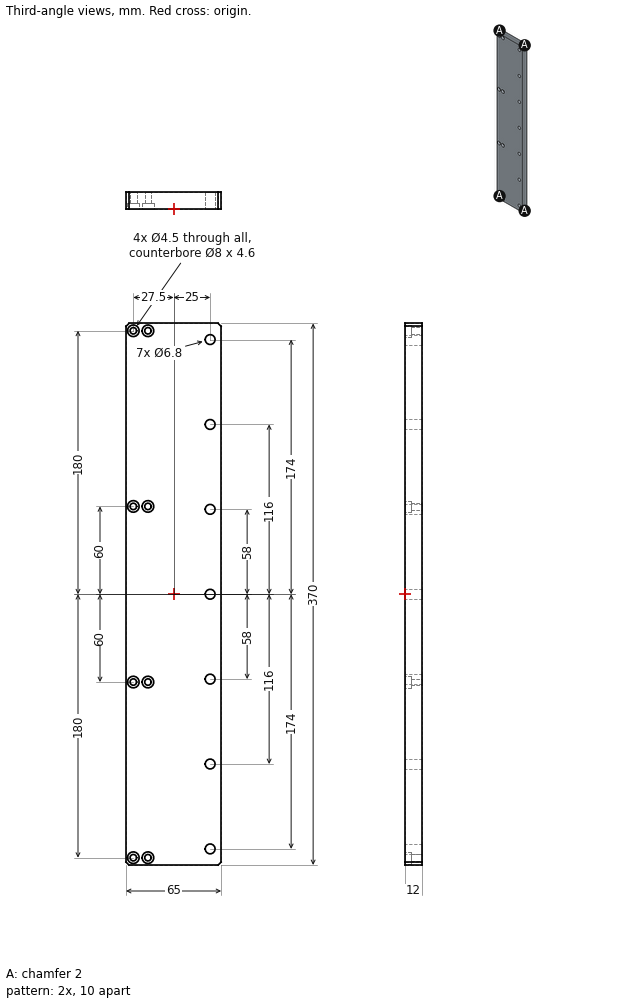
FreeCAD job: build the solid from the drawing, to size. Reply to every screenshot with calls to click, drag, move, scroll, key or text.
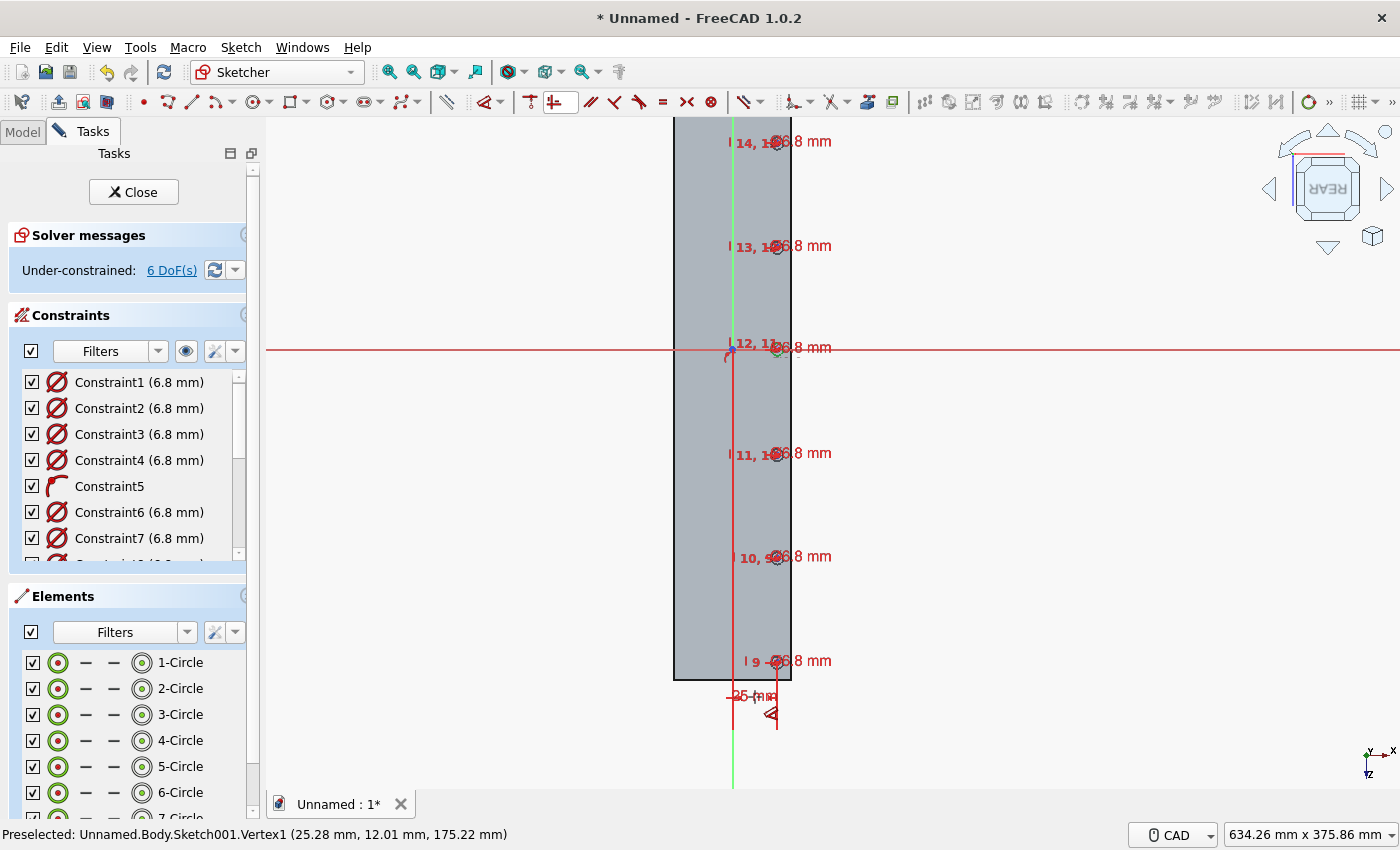
click(777, 455)
click(699, 402)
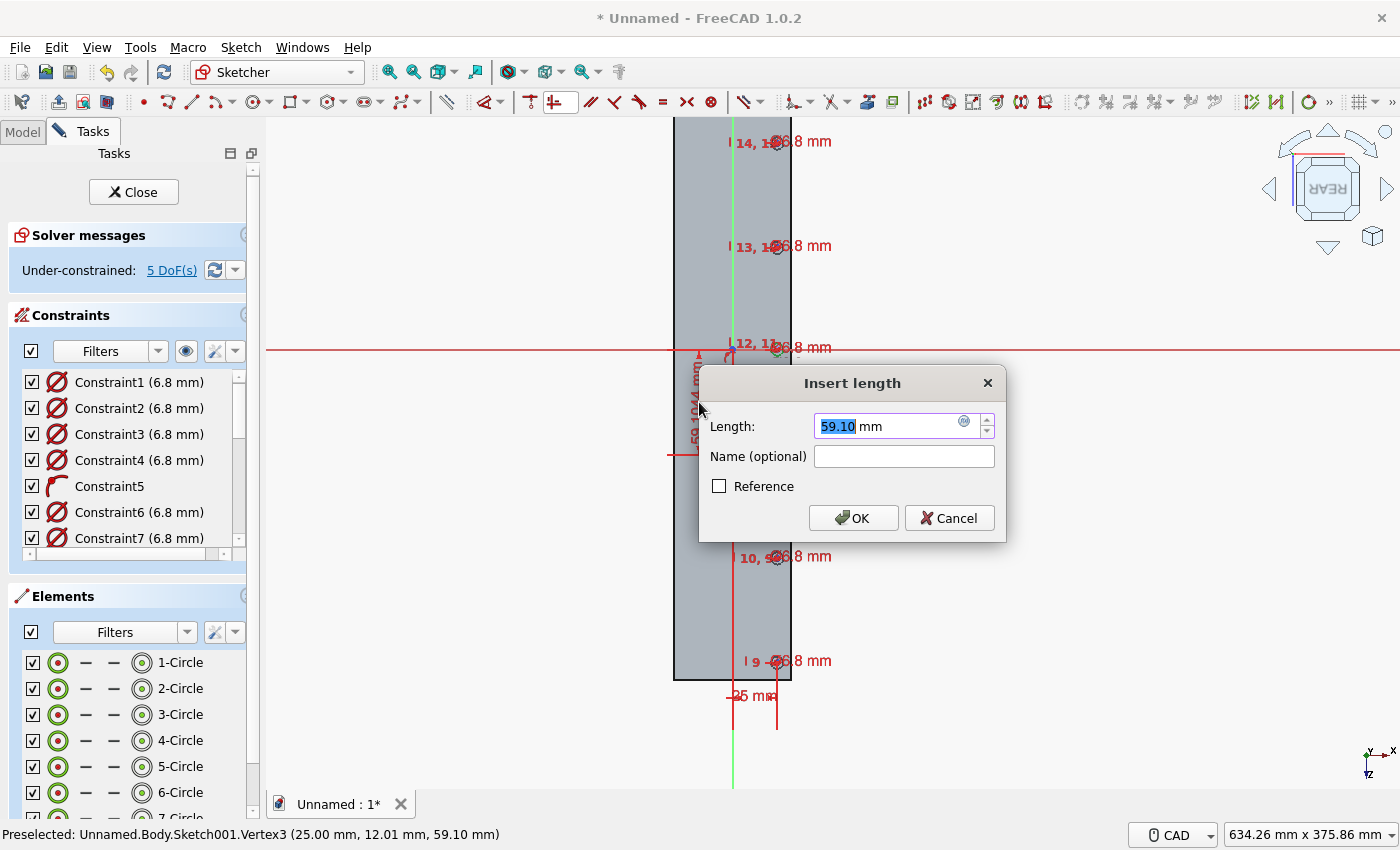
text(58)
key(Return)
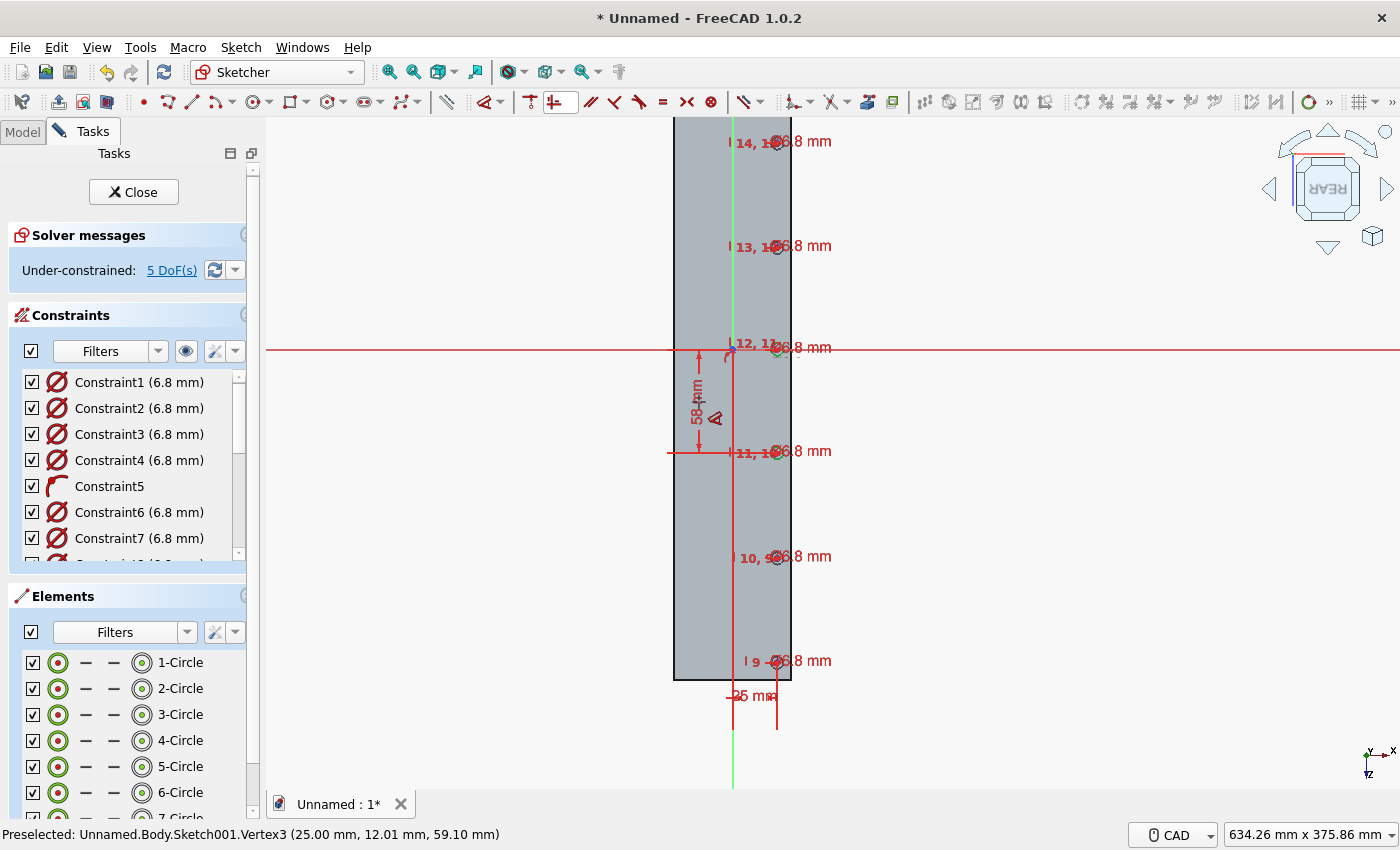
click(777, 248)
click(699, 299)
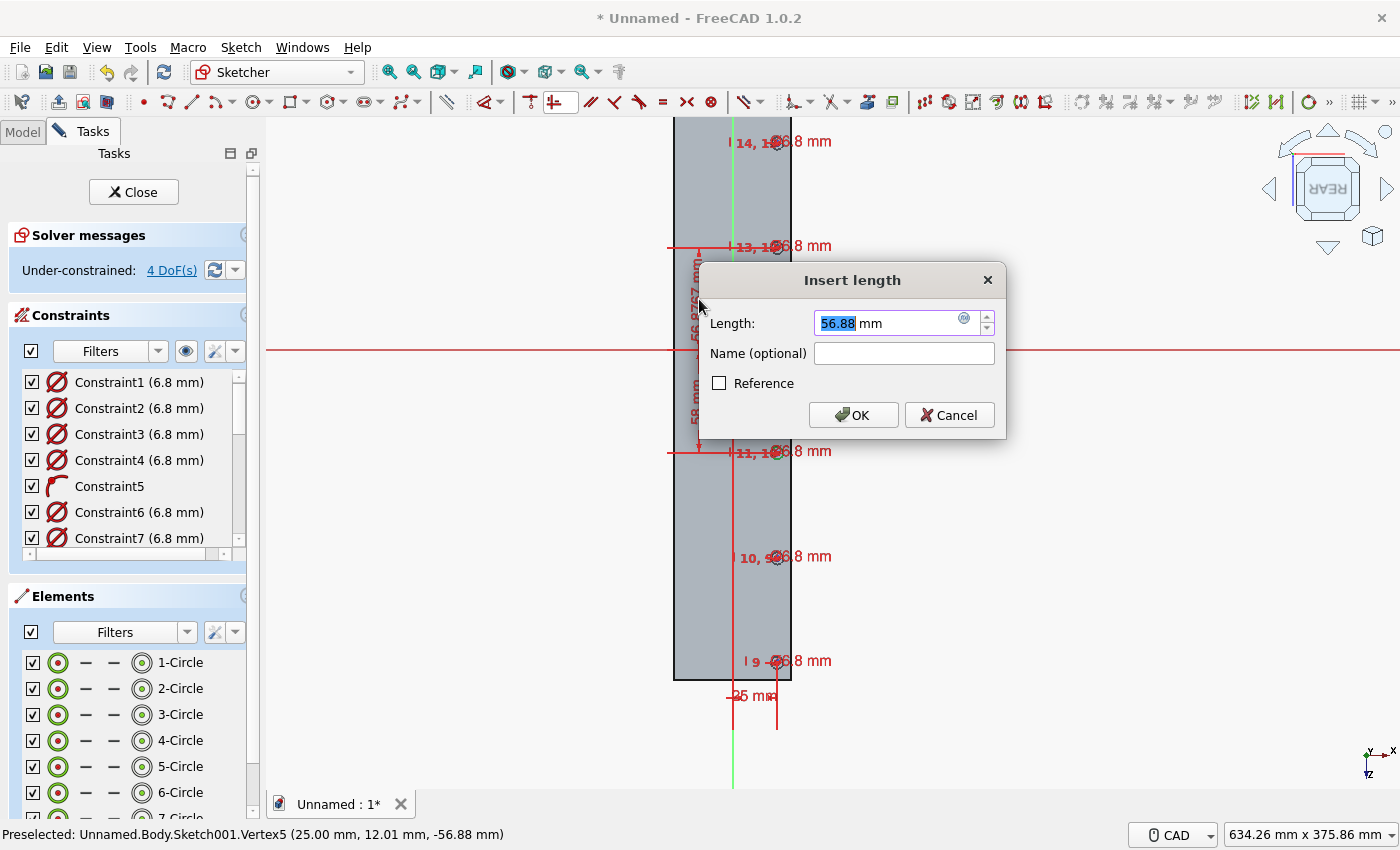
text(58)
key(Return)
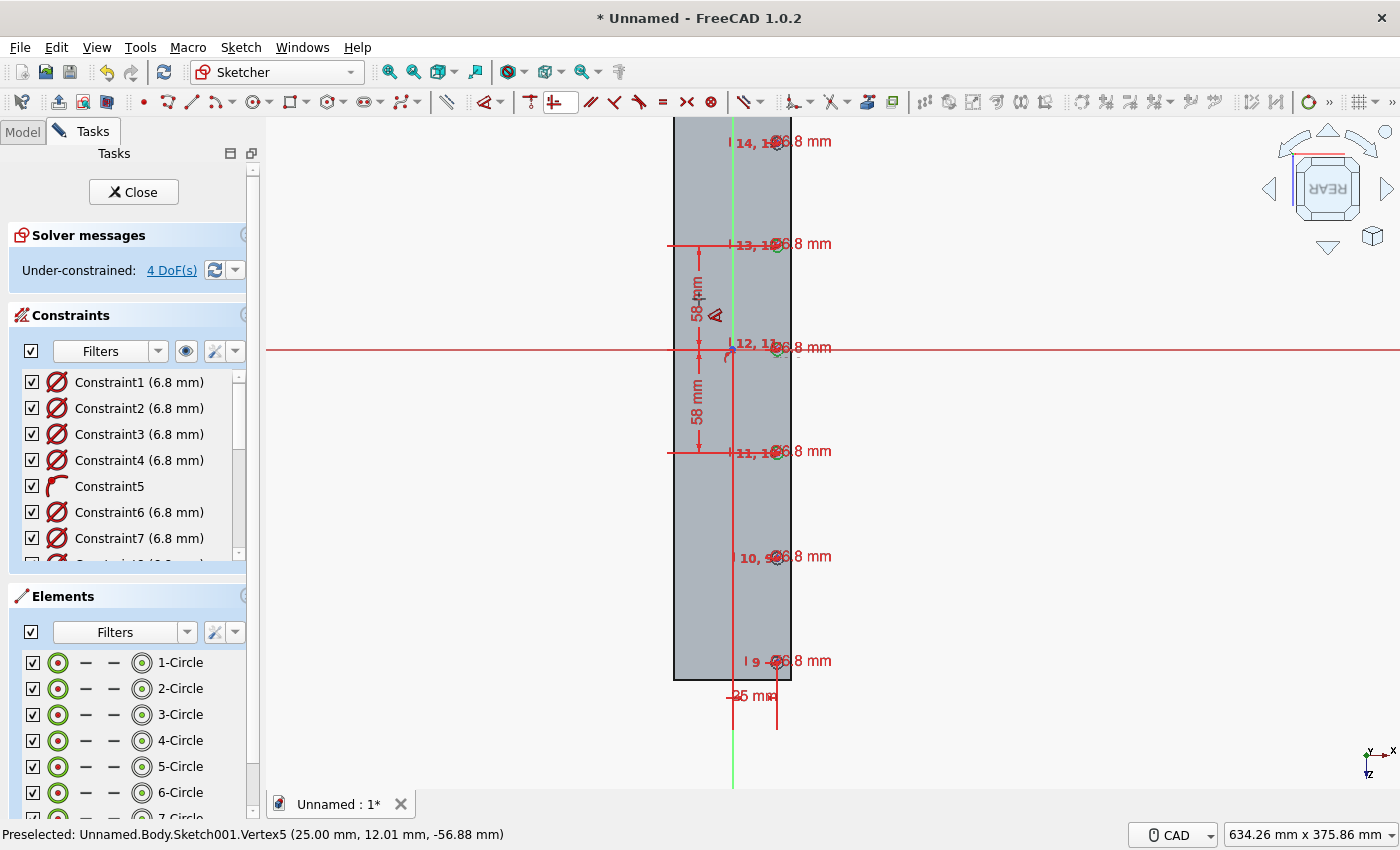
click(777, 663)
click(699, 506)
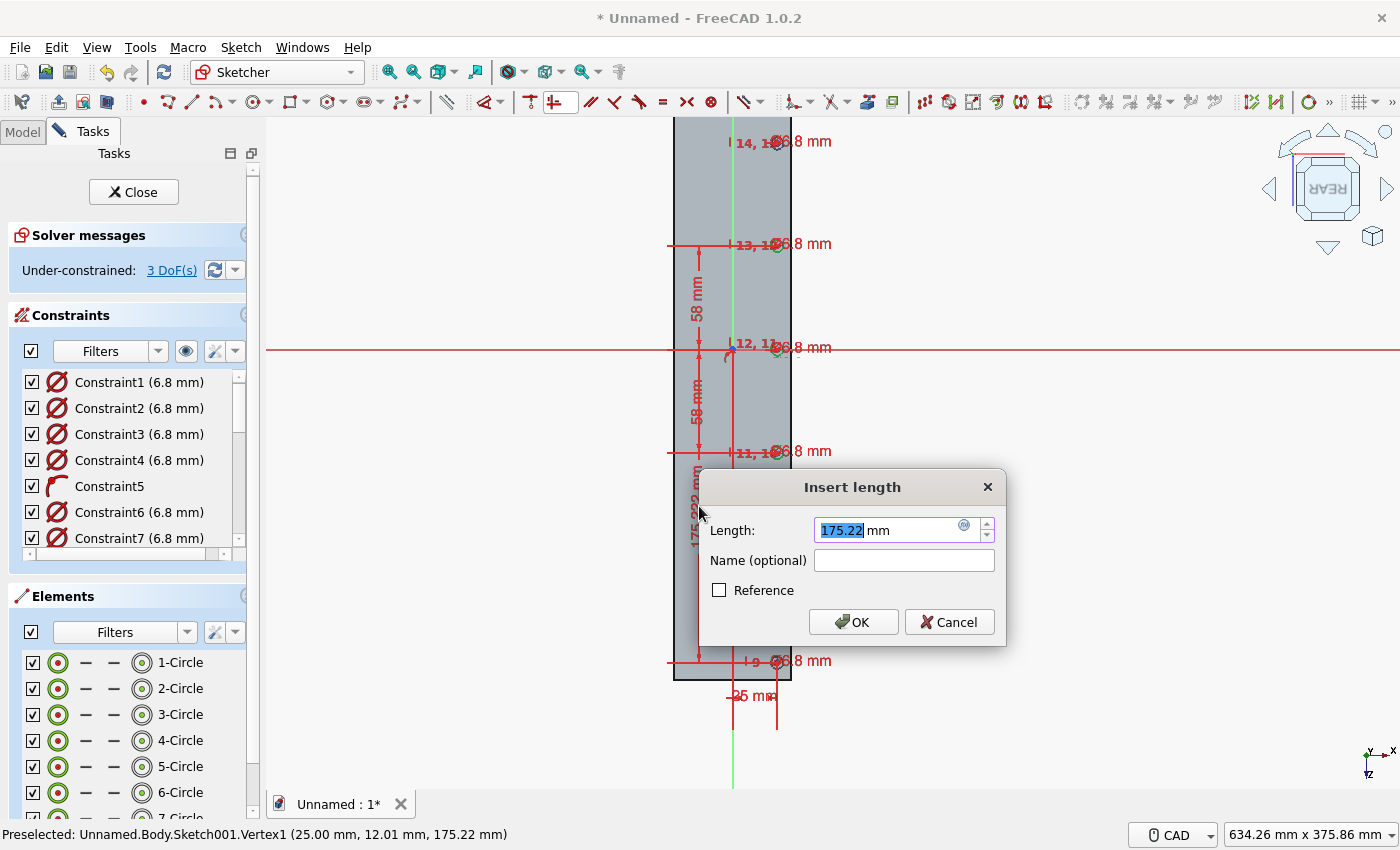
text(174)
key(Return)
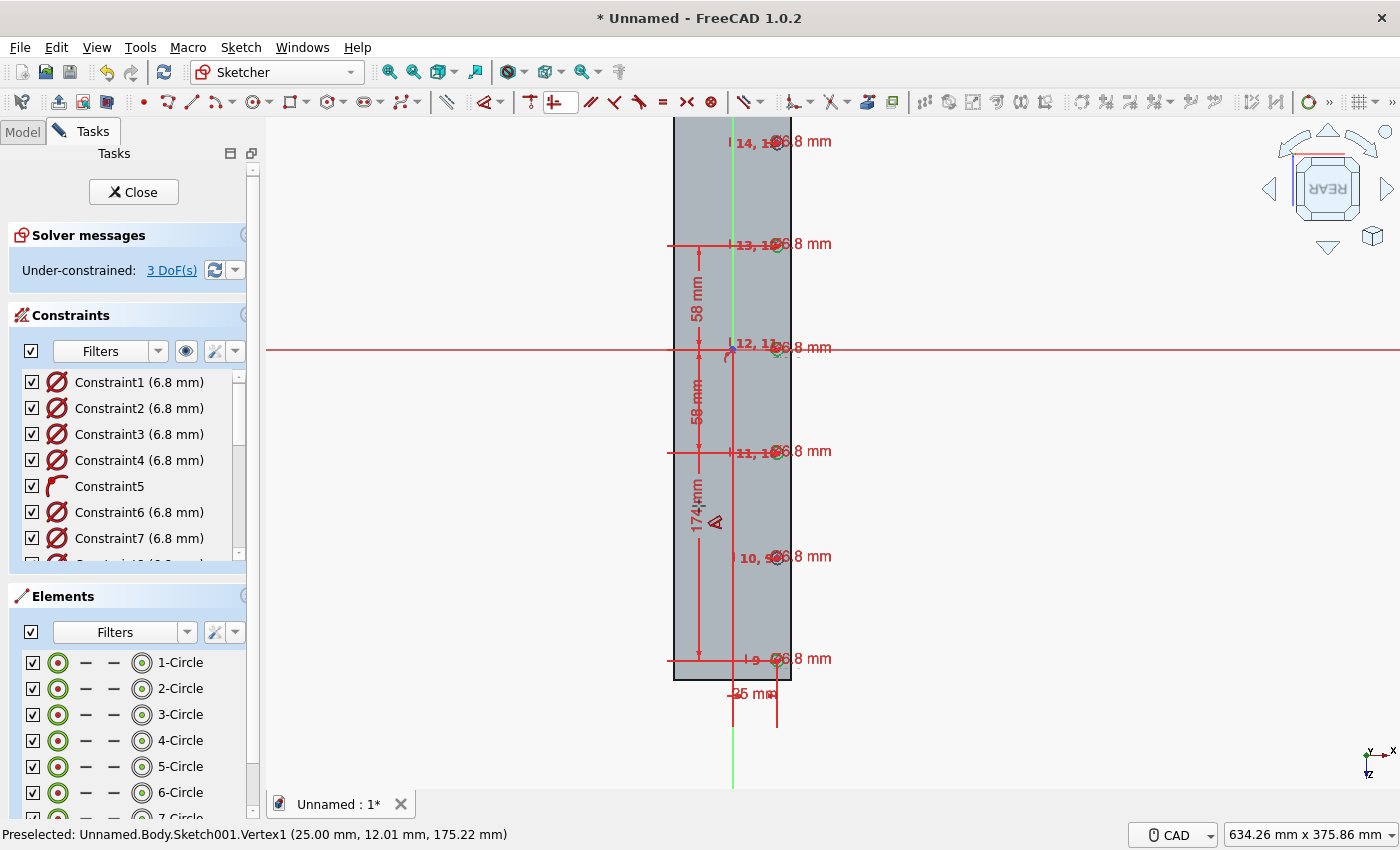
click(777, 558)
click(699, 454)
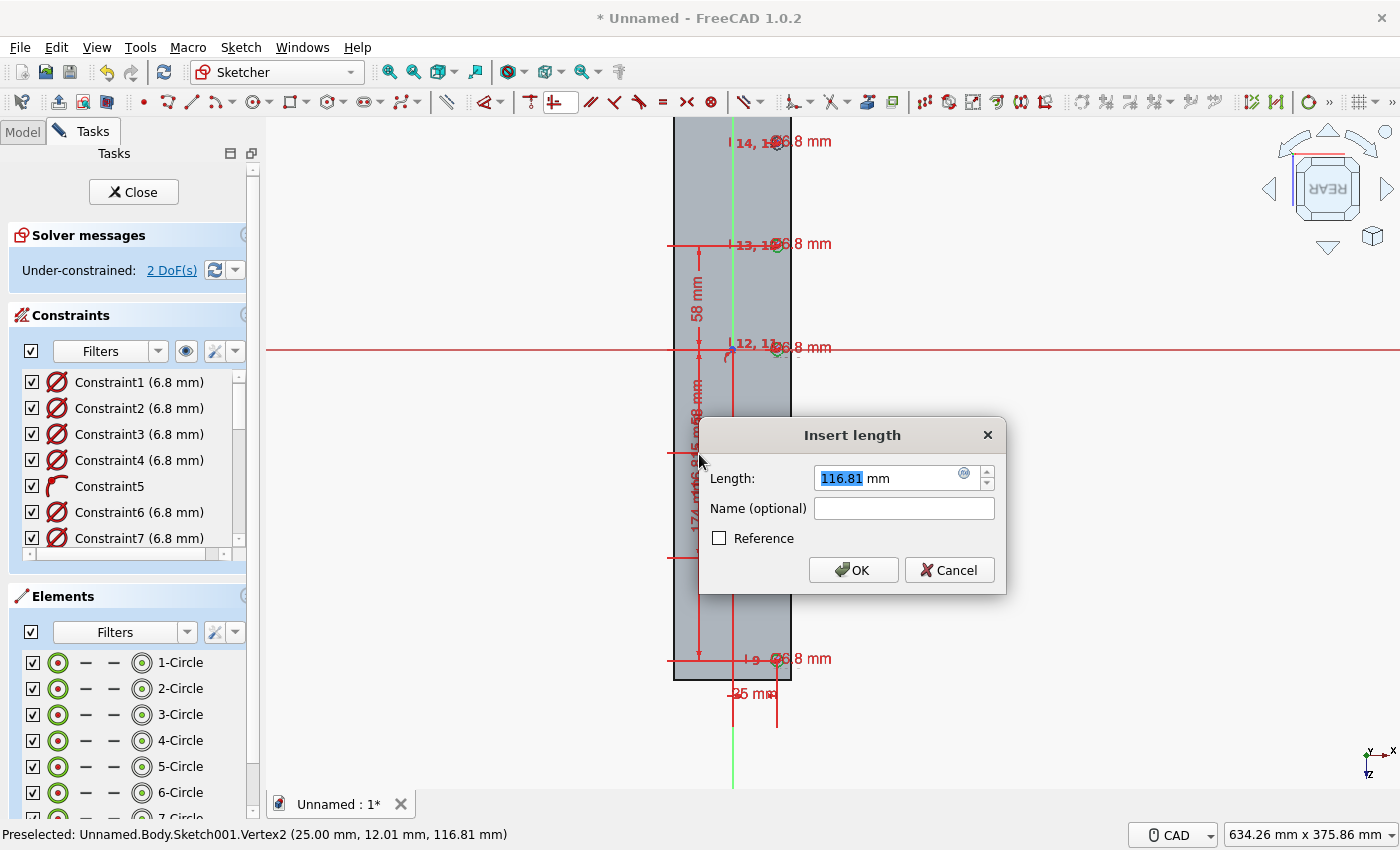
text(116)
key(Return)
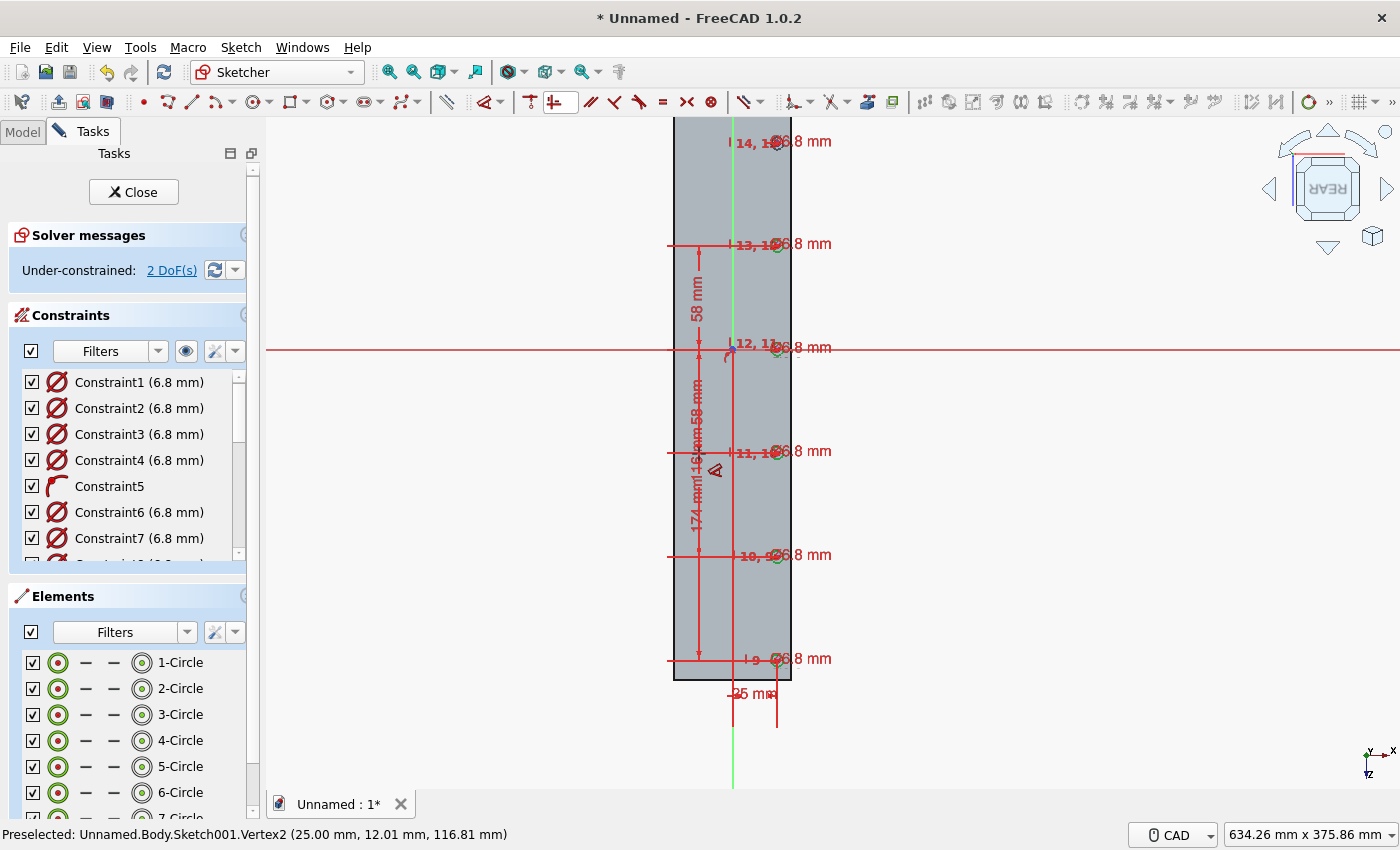
scroll(778, 663, down, 2)